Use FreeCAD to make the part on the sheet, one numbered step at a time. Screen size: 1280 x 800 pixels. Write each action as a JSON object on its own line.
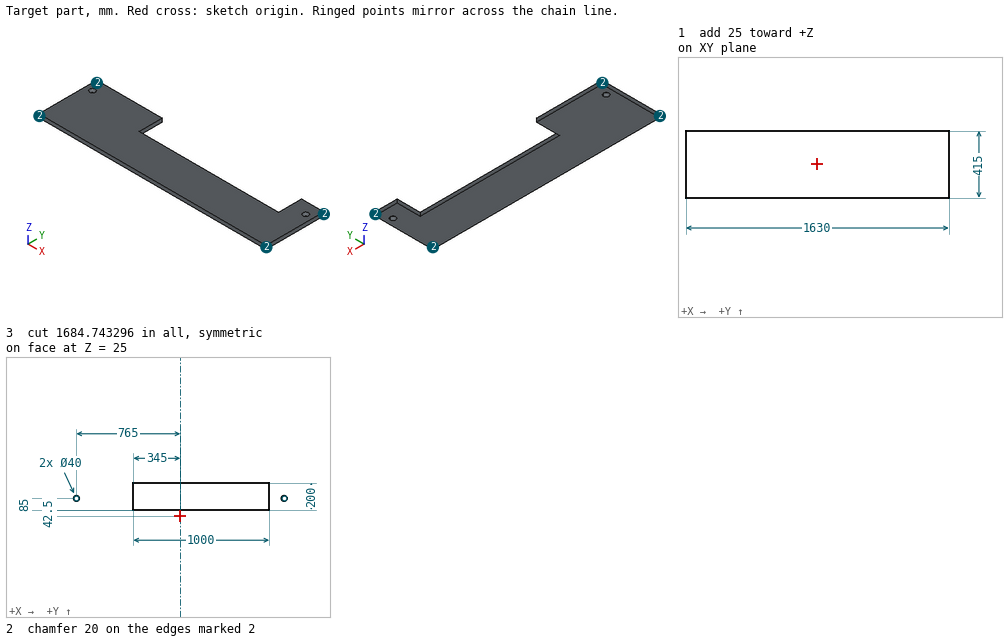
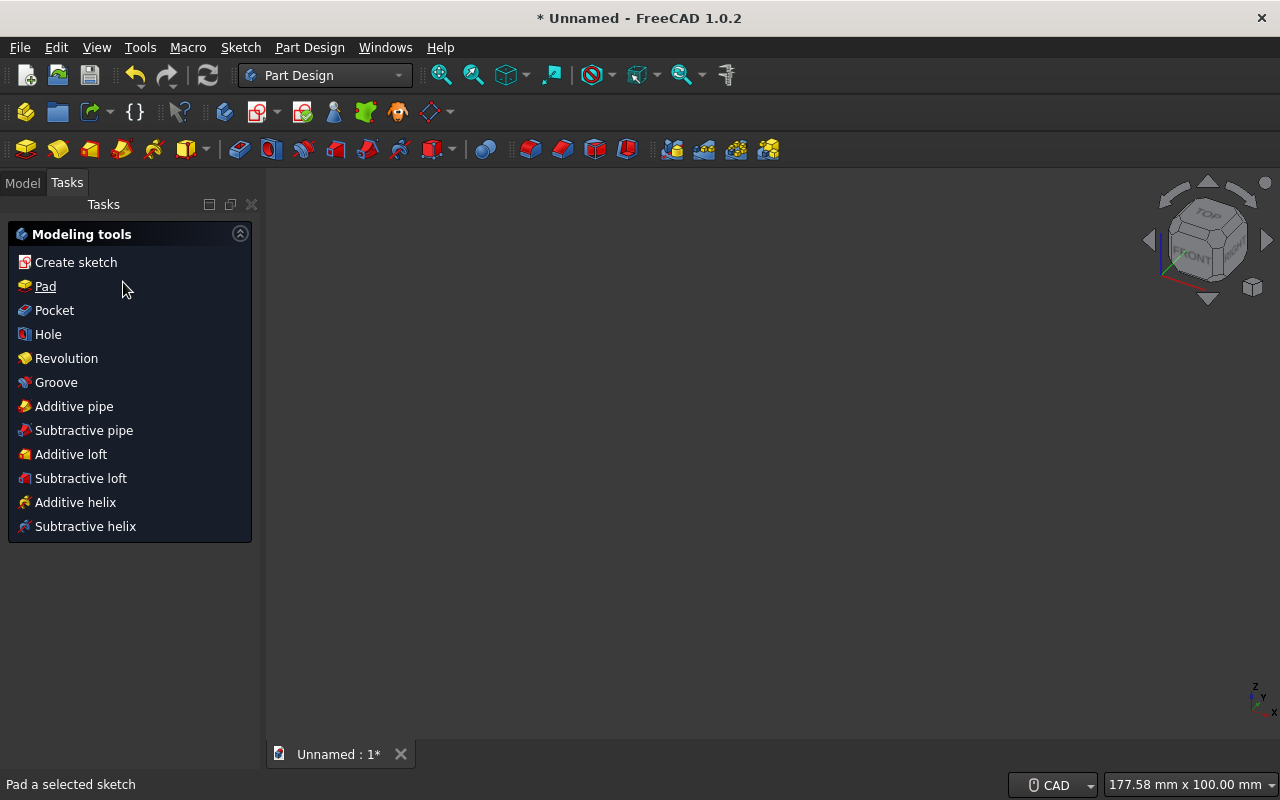
{"action": "left_click", "coordinate": [26, 150]}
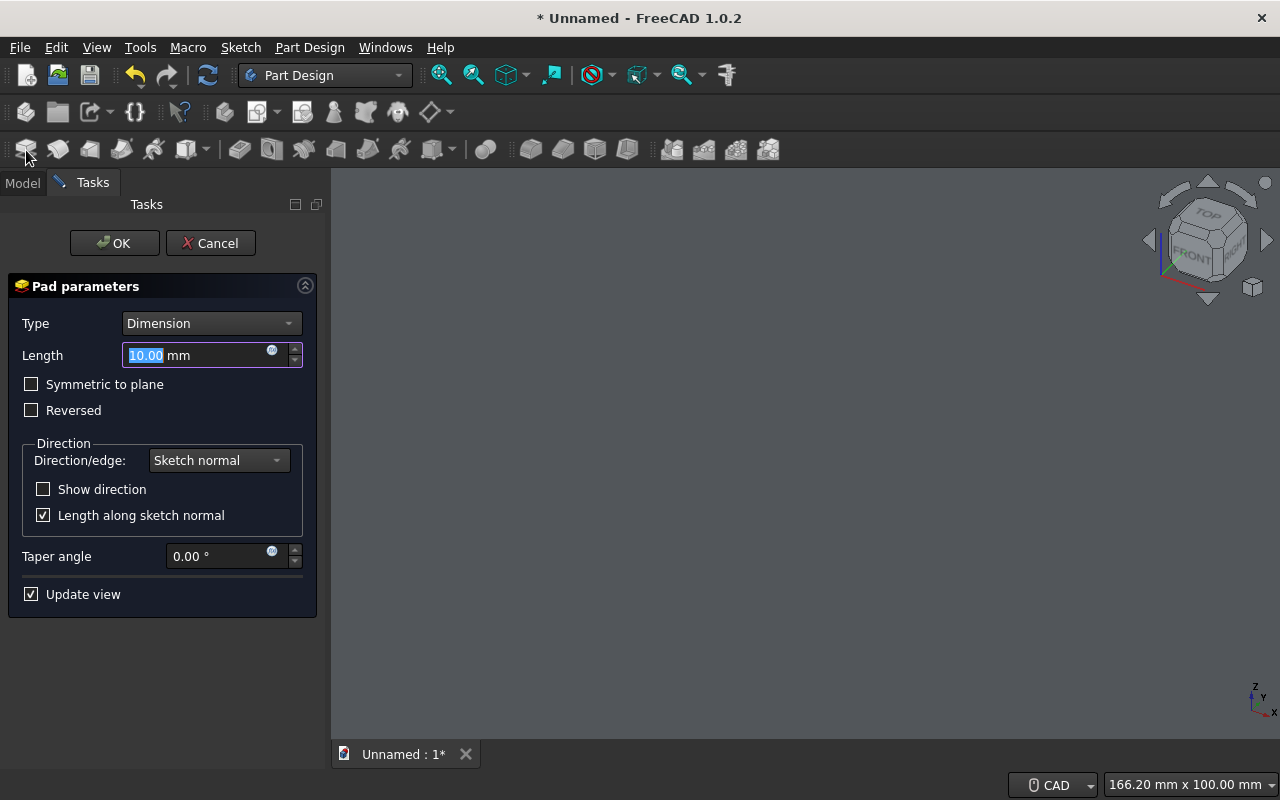
{"action": "type", "text": "25"}
{"action": "key", "text": "Tab"}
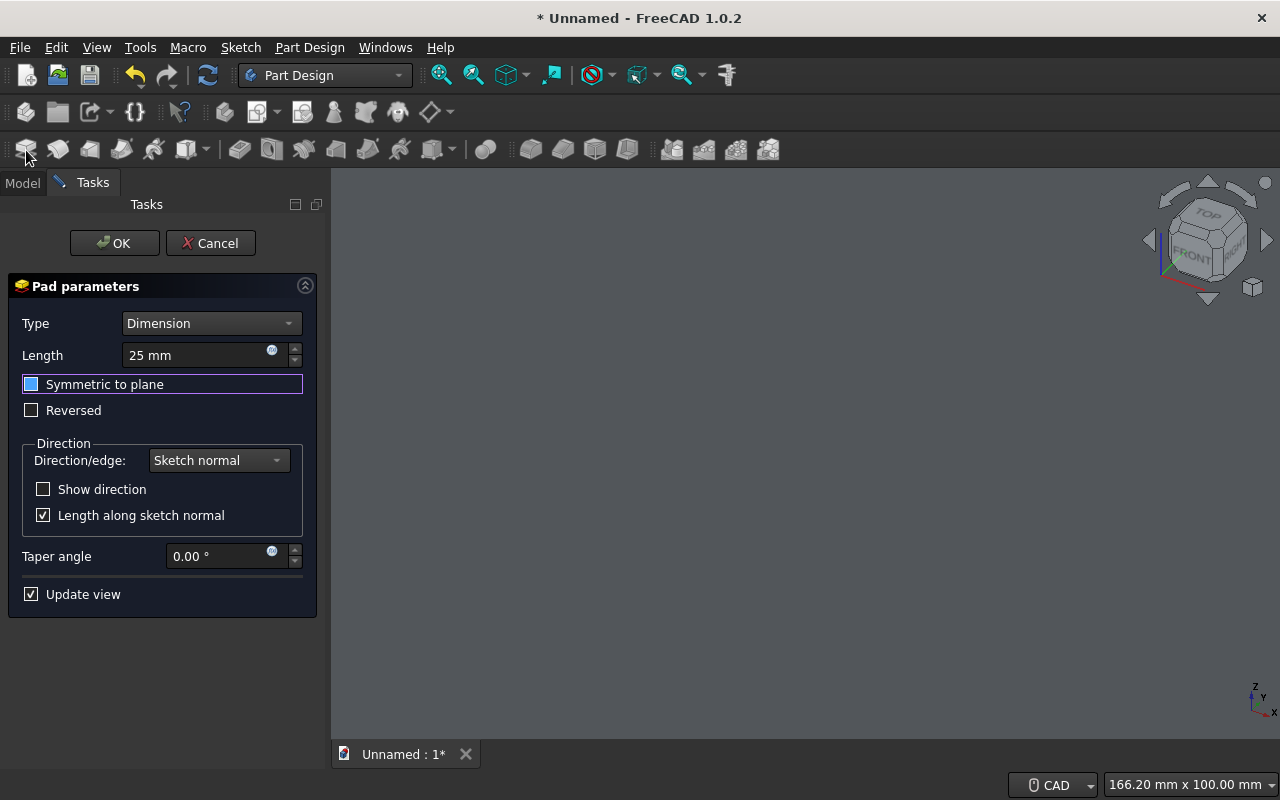
{"action": "left_click", "coordinate": [115, 243]}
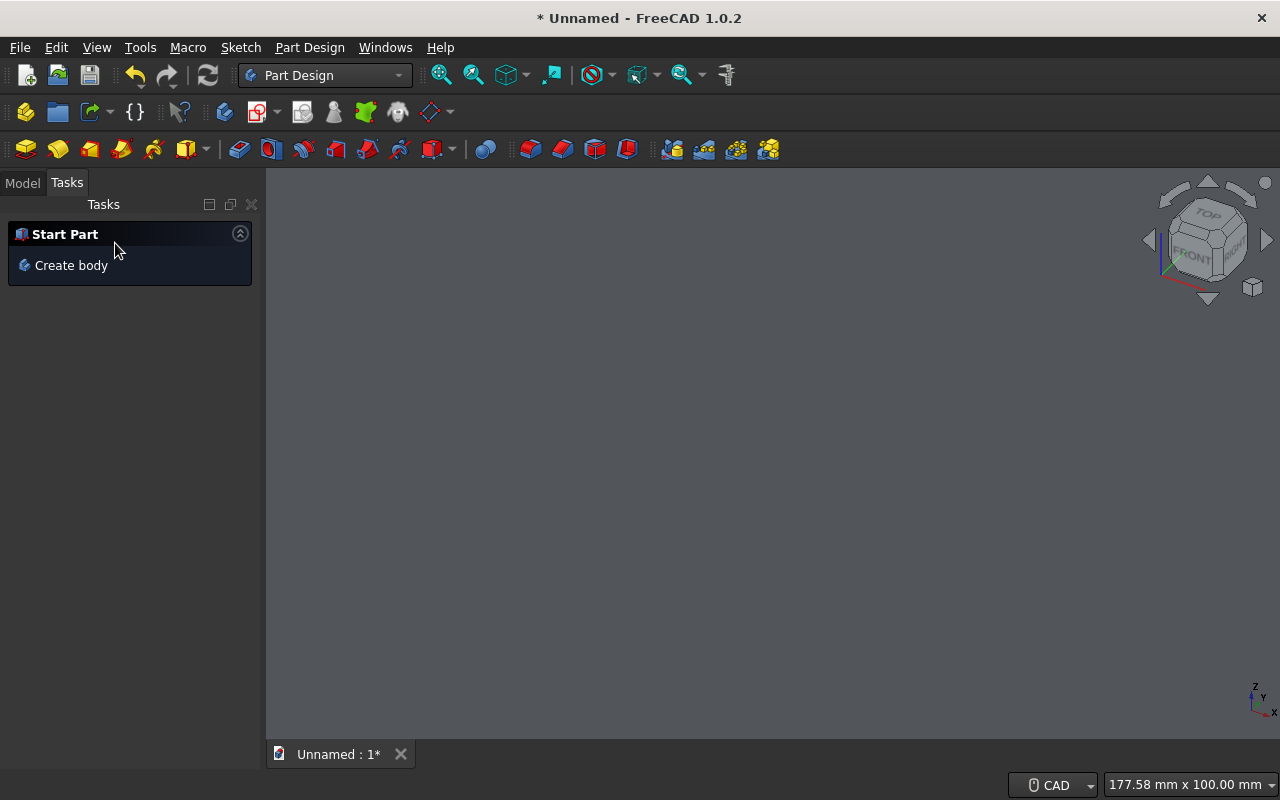
{"action": "key", "text": "v f"}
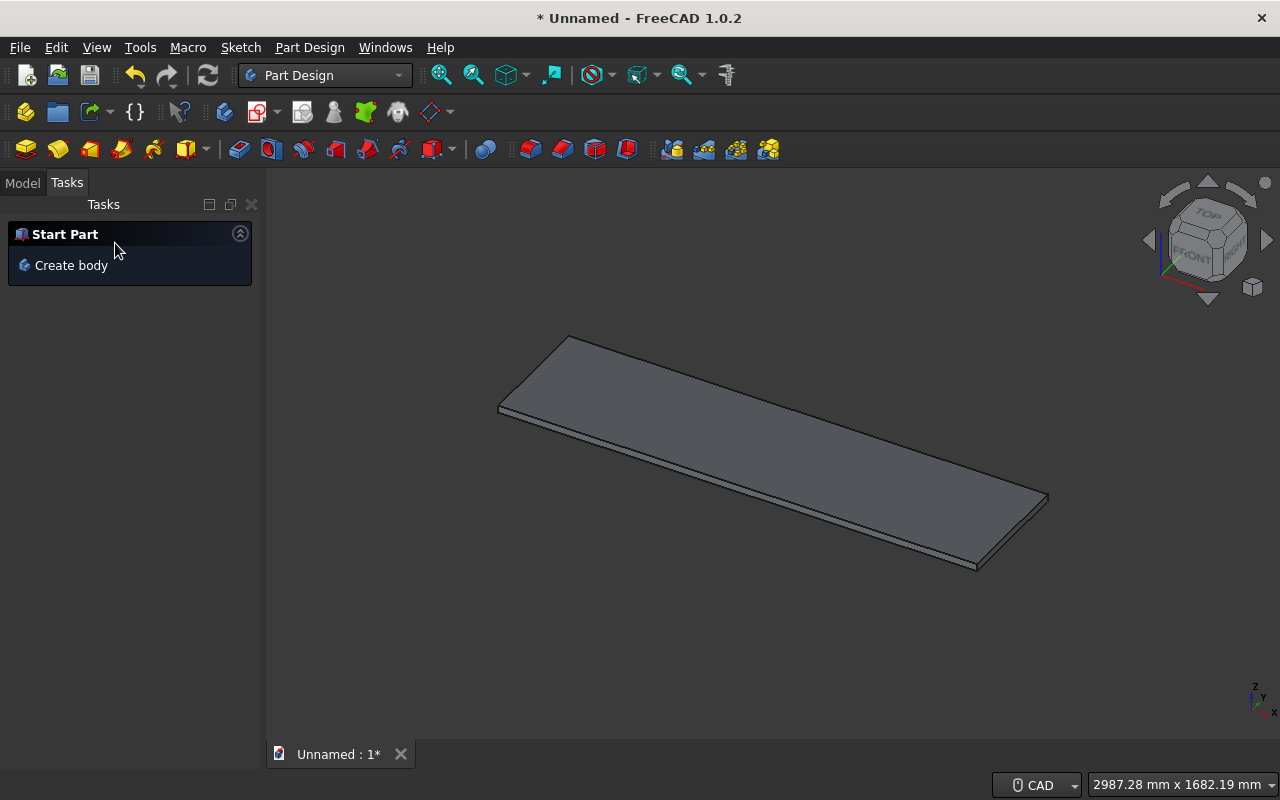
{"action": "scroll", "coordinate": [569, 338], "scroll_direction": "up", "scroll_amount": 8}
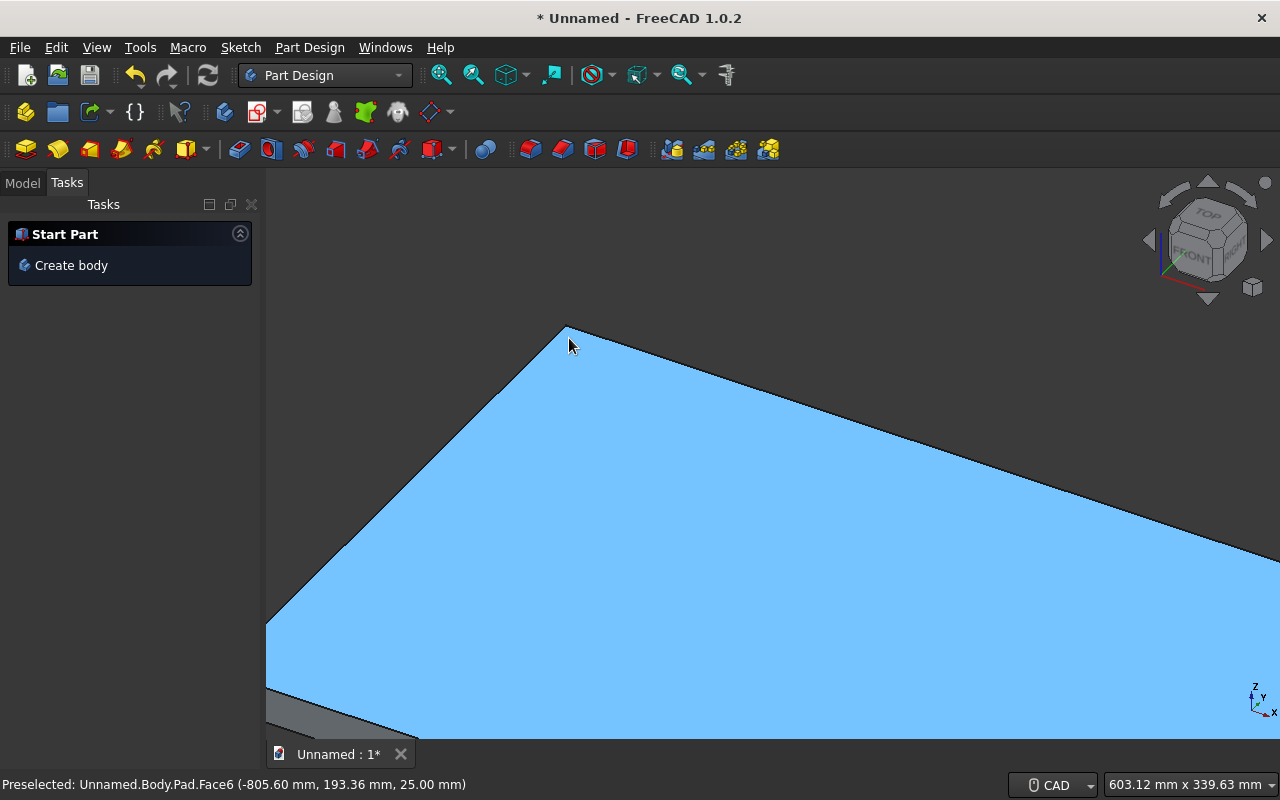
{"action": "left_click", "coordinate": [442, 76]}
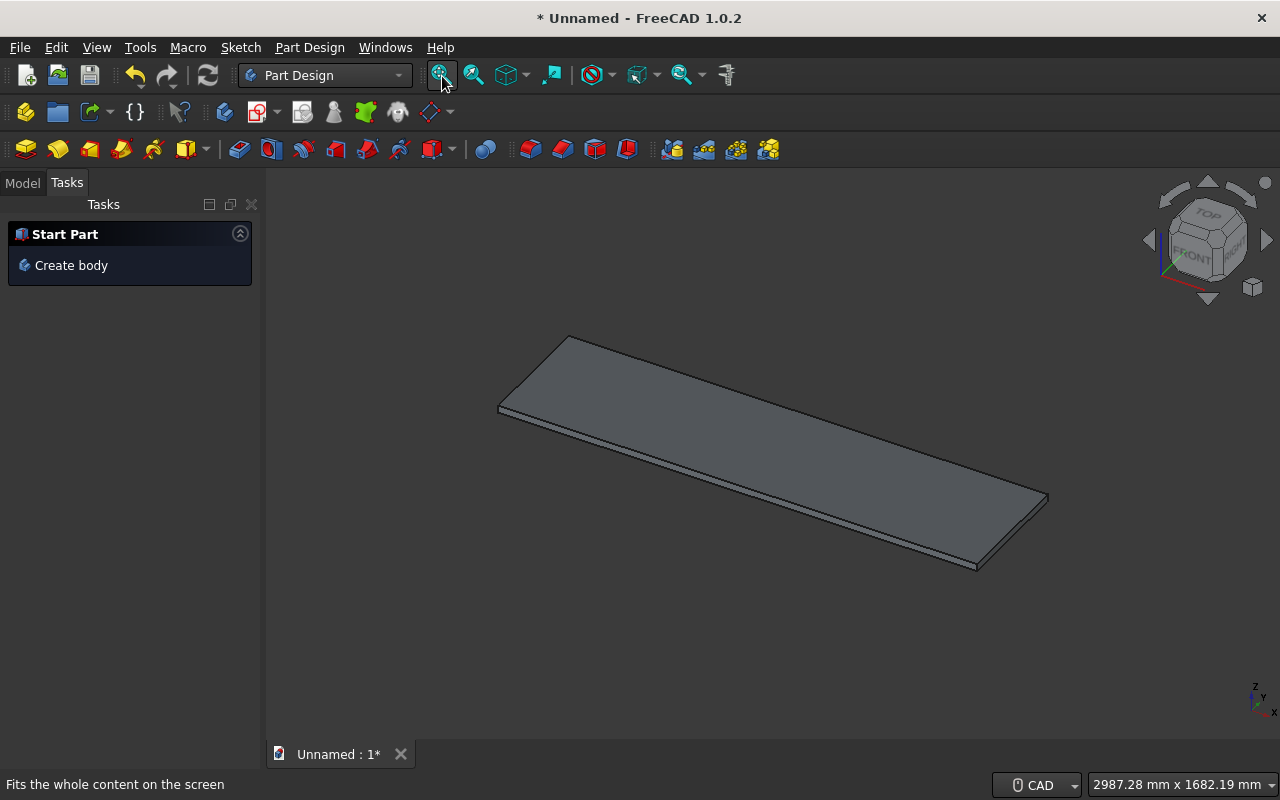
{"action": "key", "text": "0"}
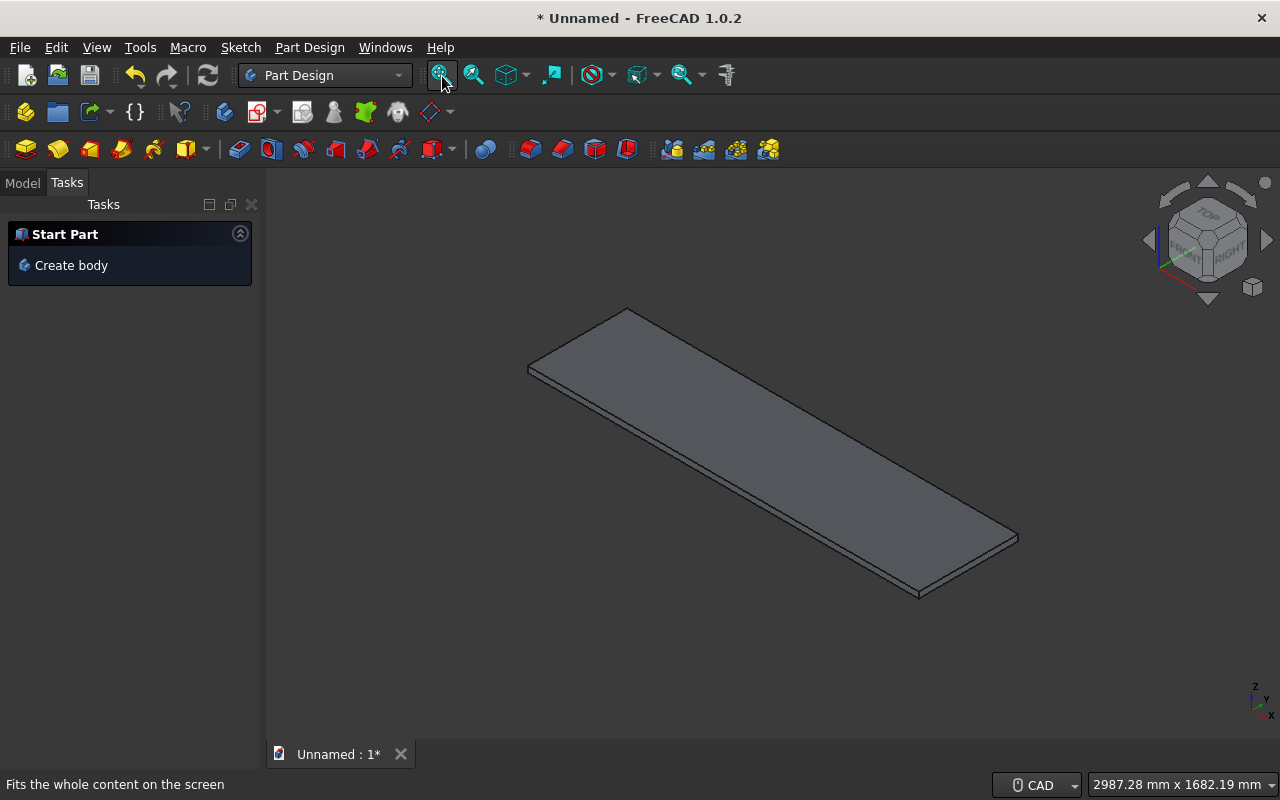
{"action": "scroll", "coordinate": [627, 311], "scroll_direction": "up", "scroll_amount": 8}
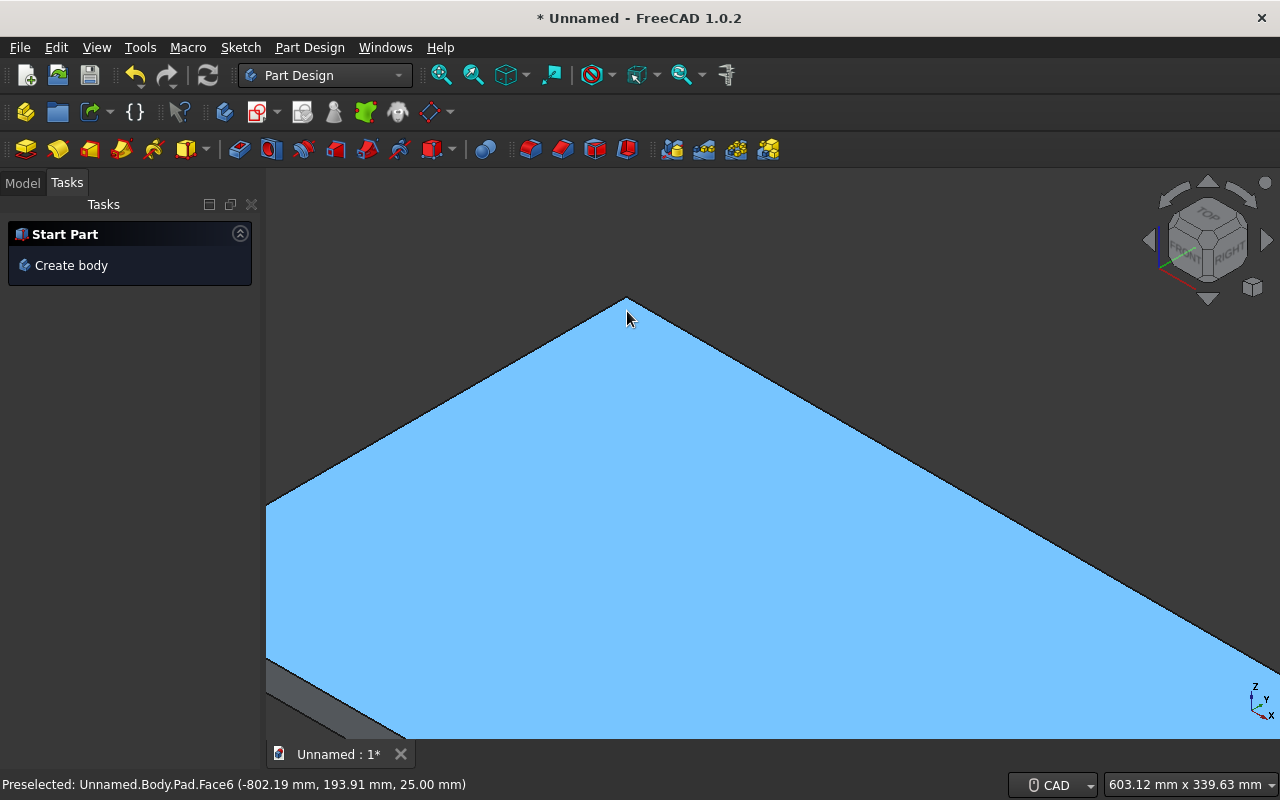
{"action": "key", "text": "v f"}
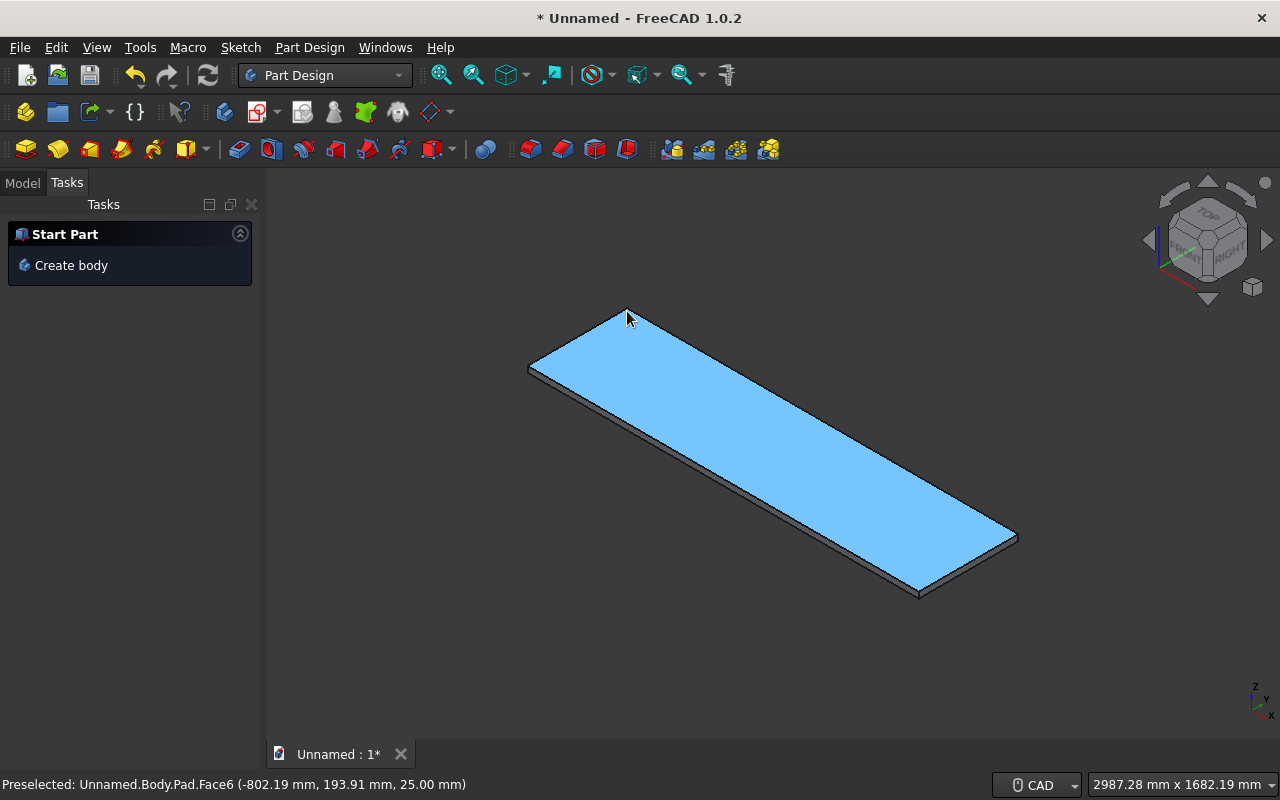
{"action": "key", "text": "2"}